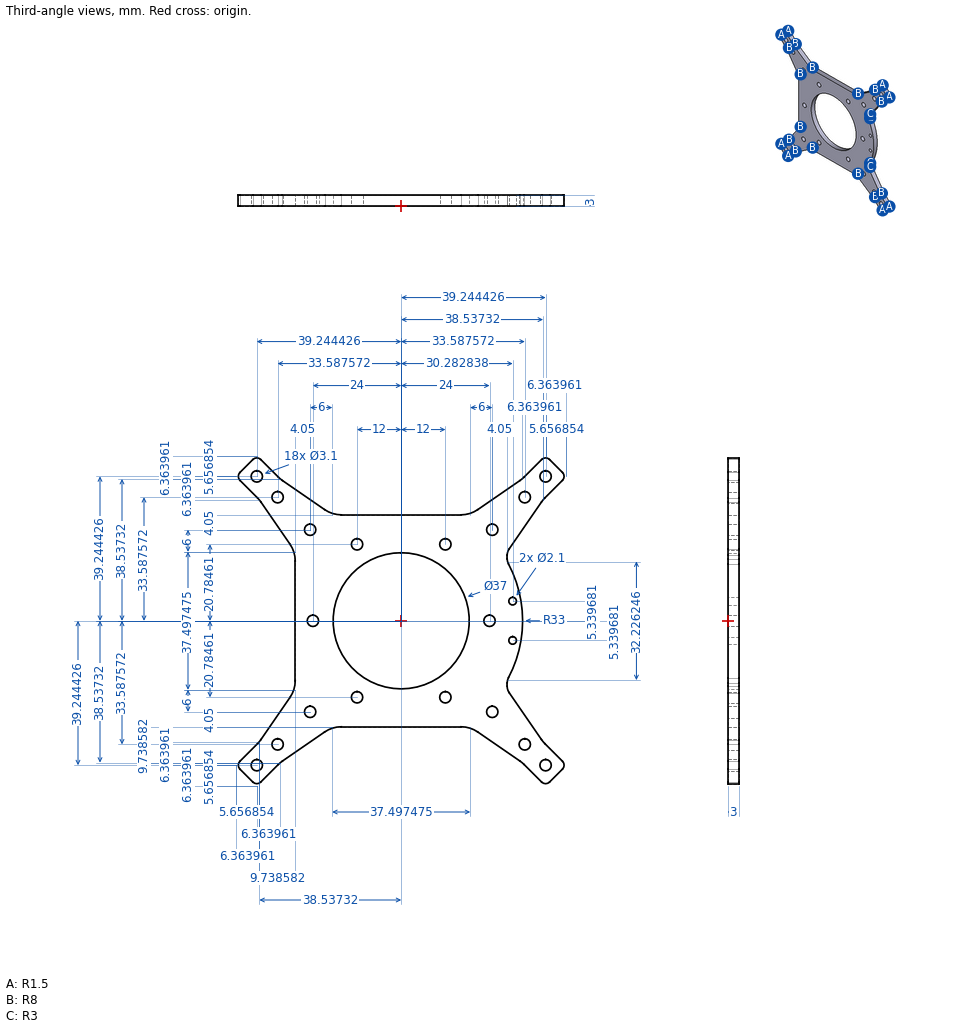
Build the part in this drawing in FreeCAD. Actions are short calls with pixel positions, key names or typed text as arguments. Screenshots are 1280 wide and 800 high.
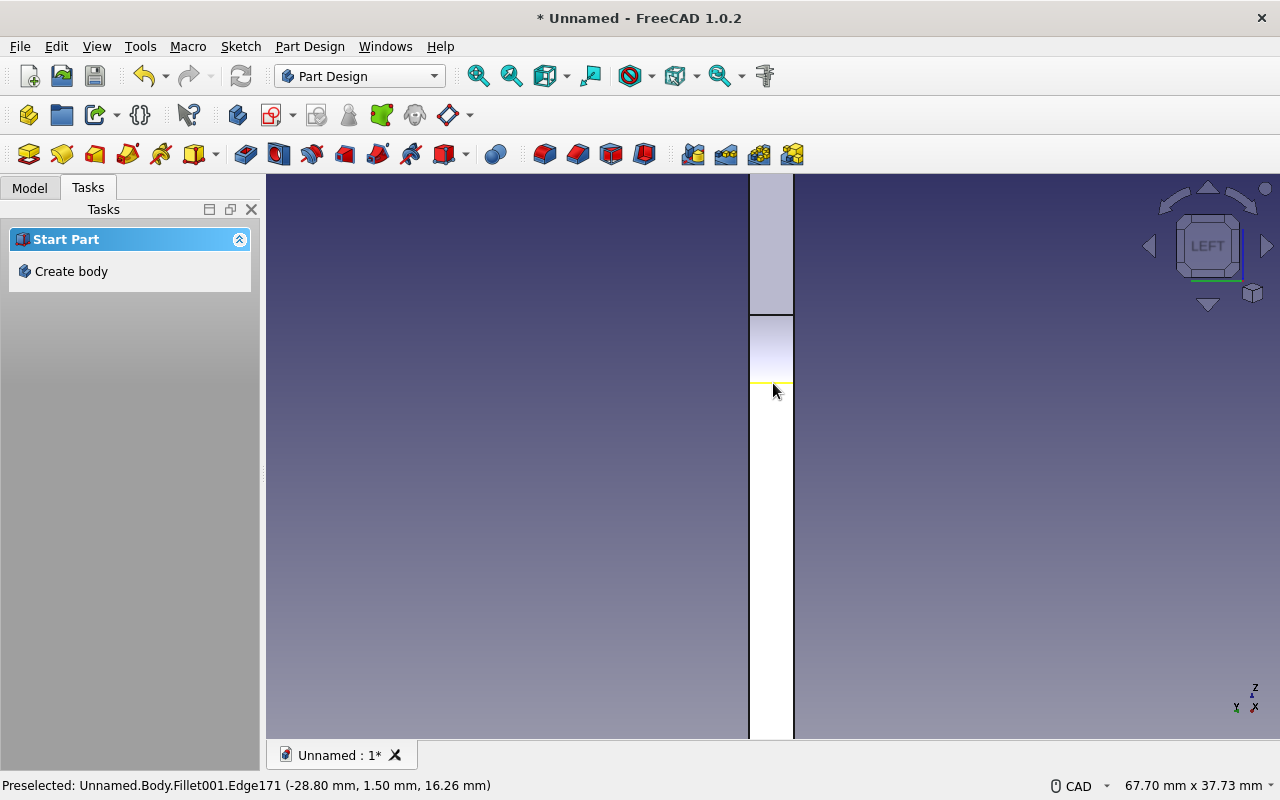
click(479, 76)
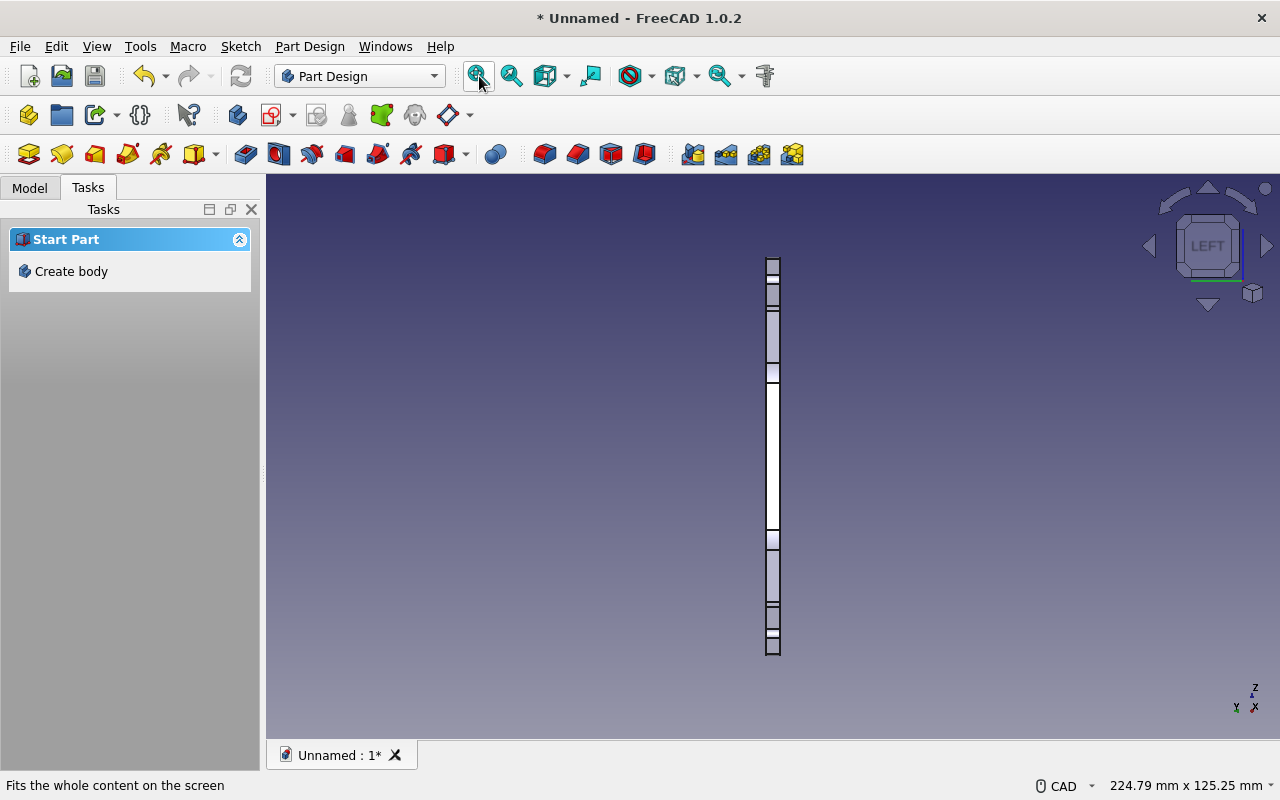
key(0)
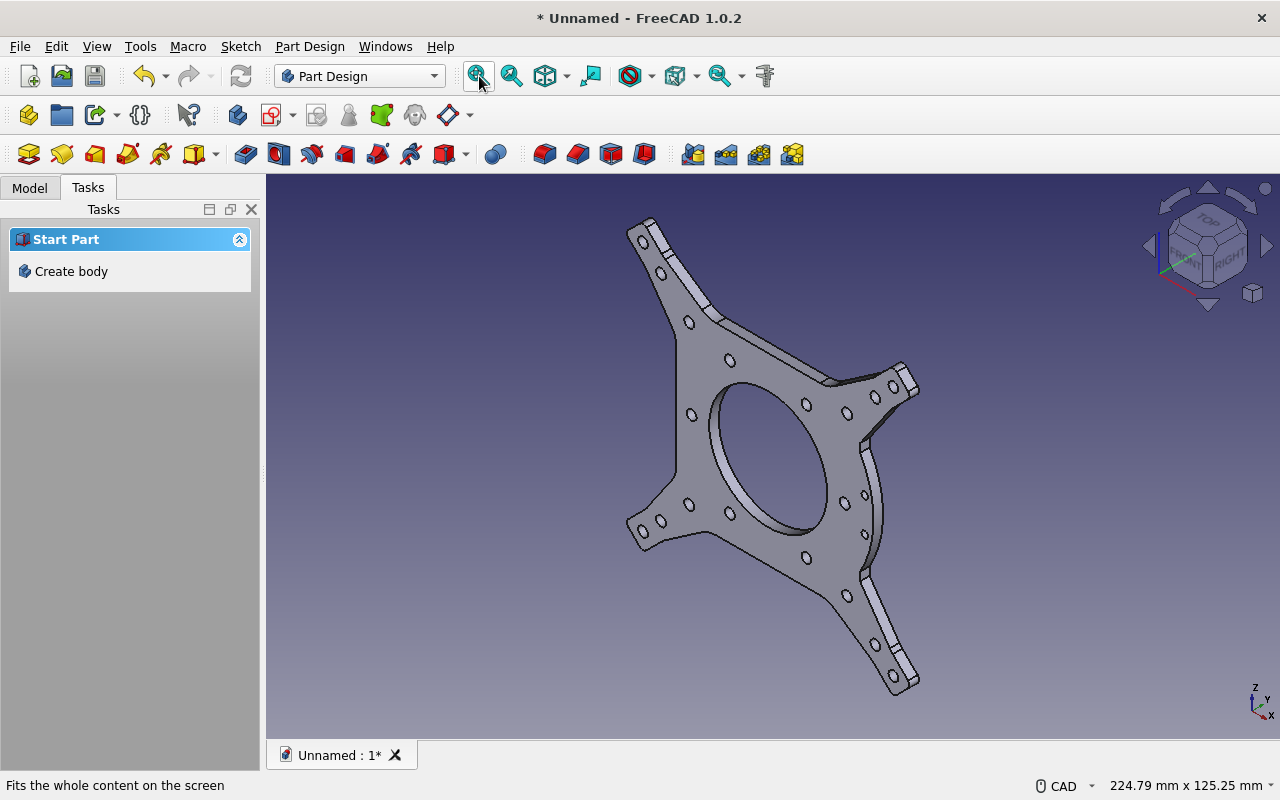
scroll(865, 449, up, 6)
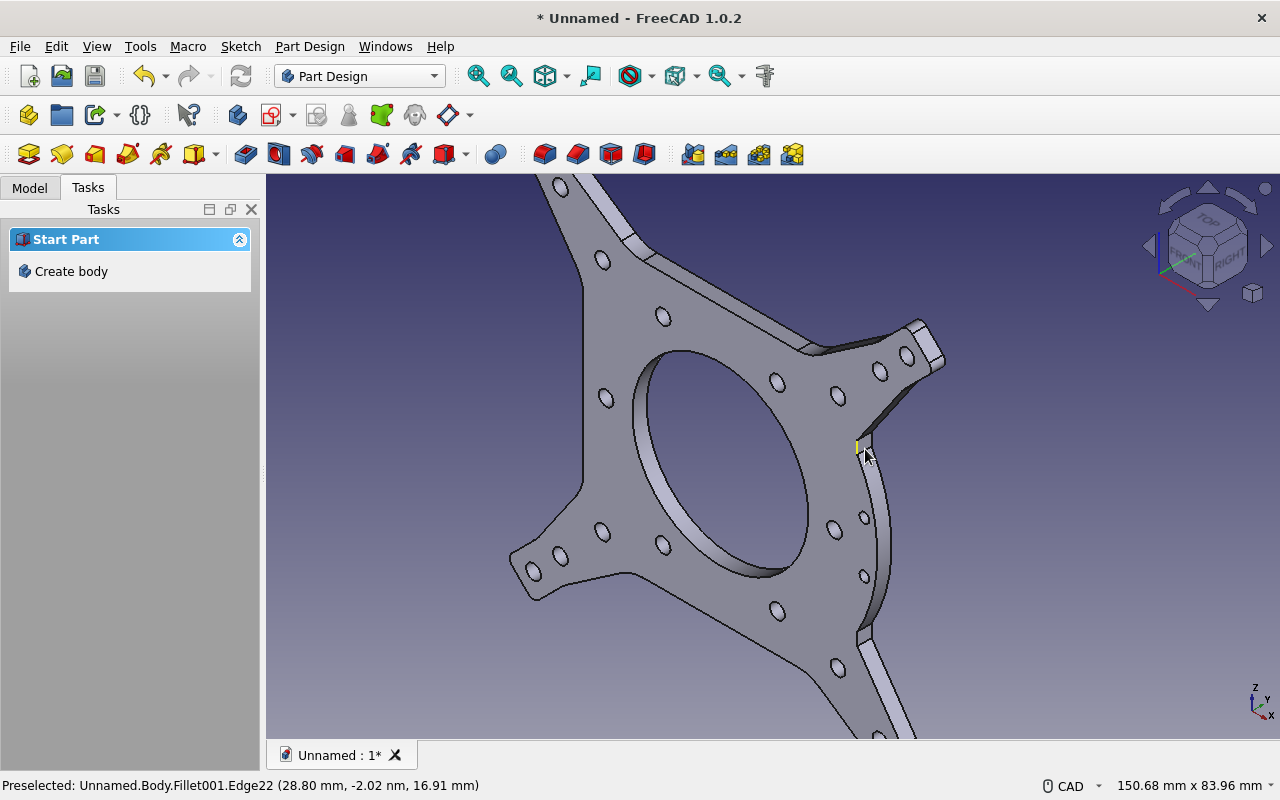
key(v)
key(f)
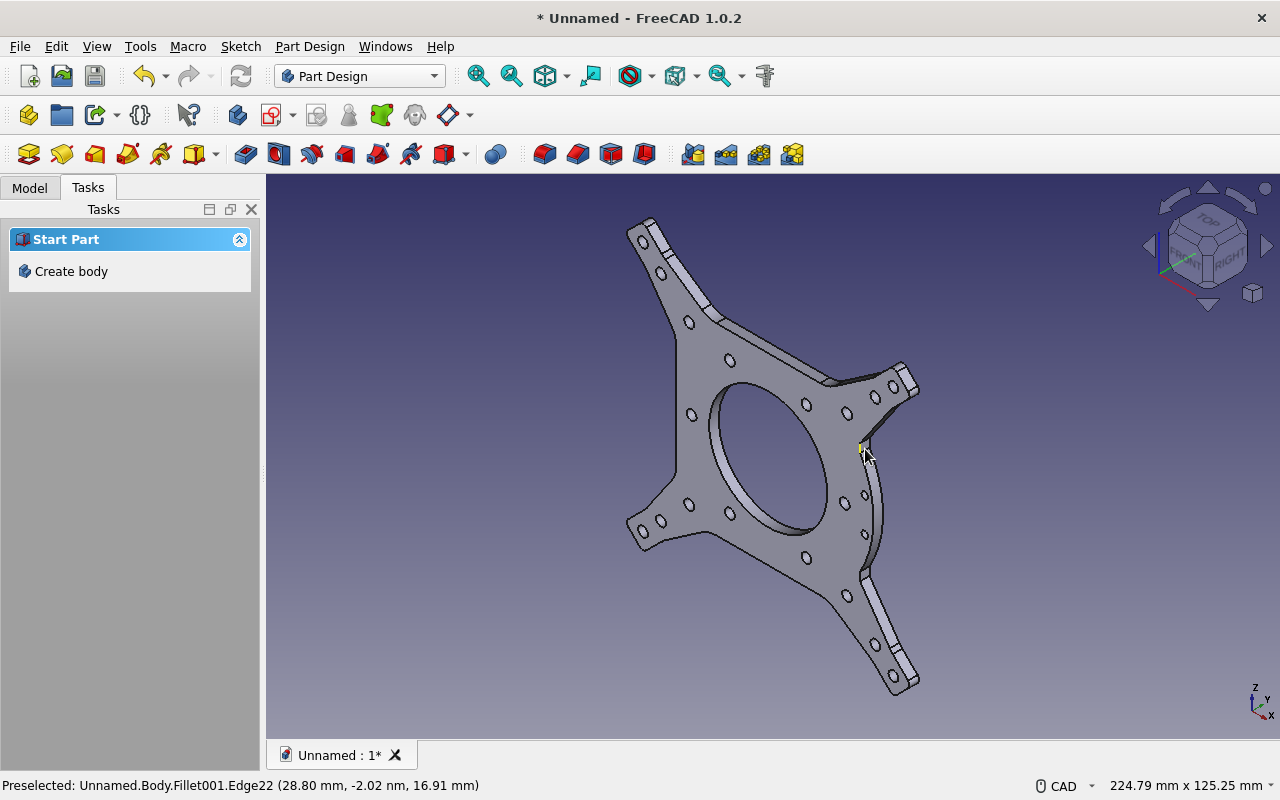
key(2)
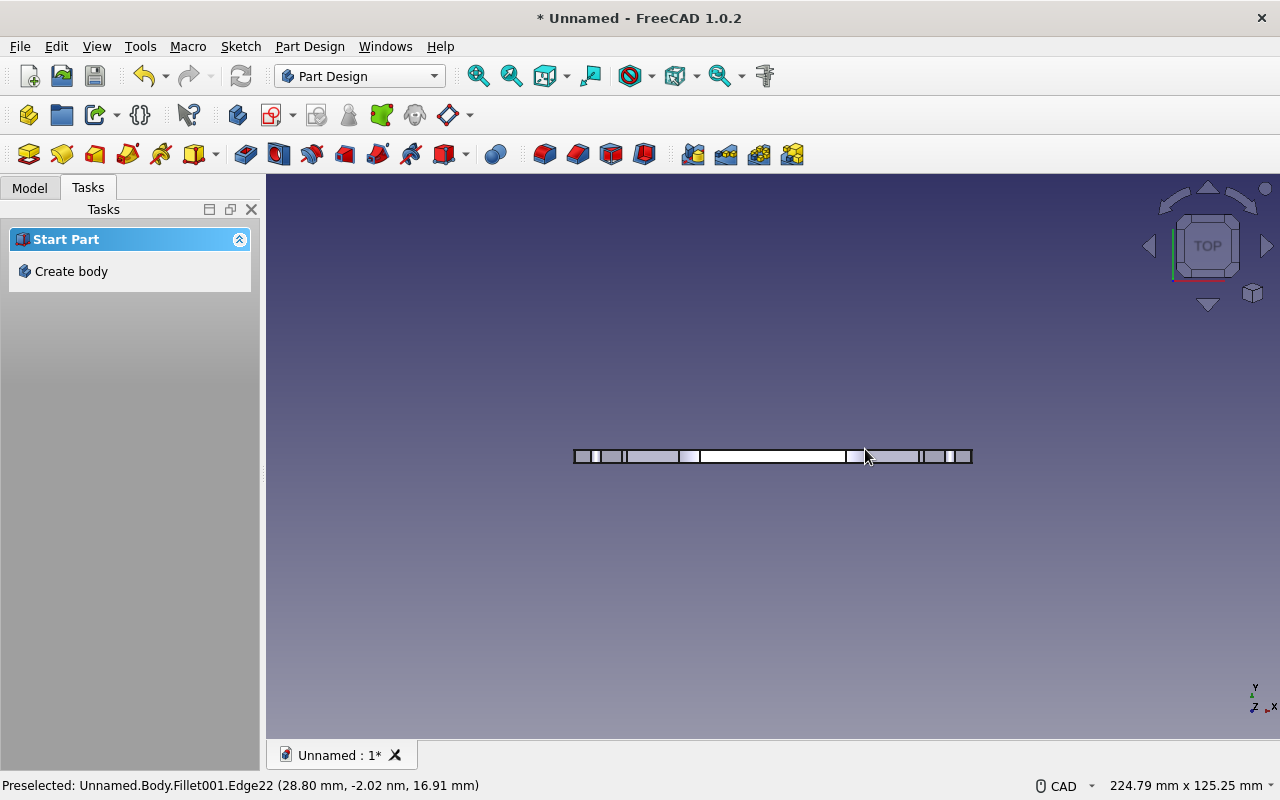
click(479, 76)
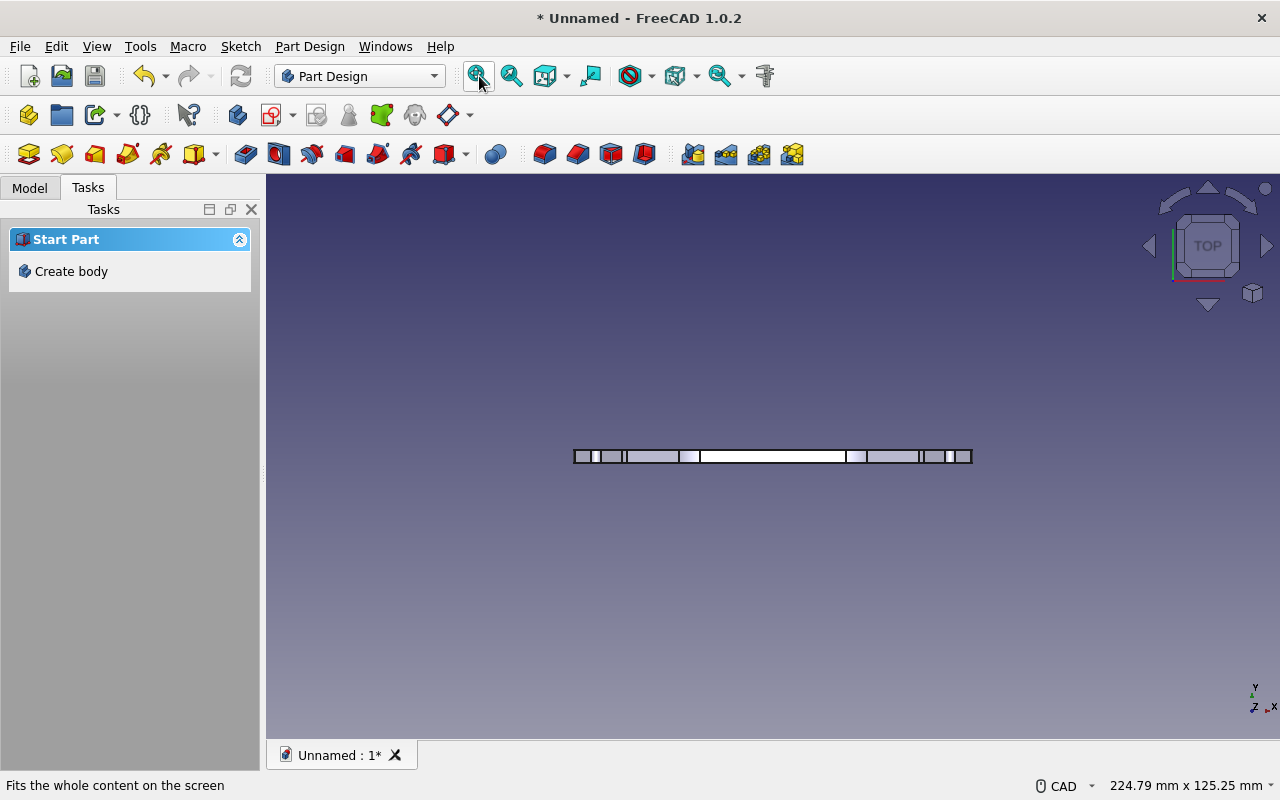
scroll(903, 455, up, 6)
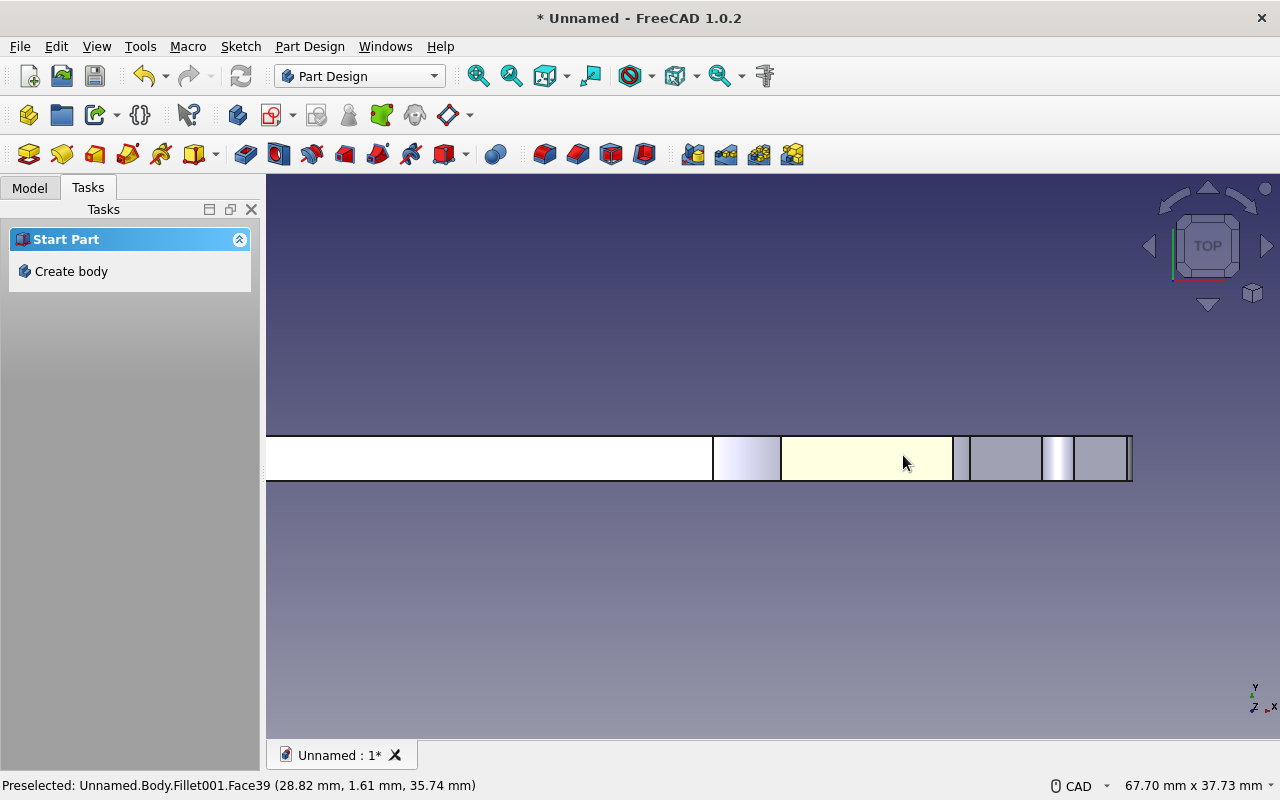
click(479, 76)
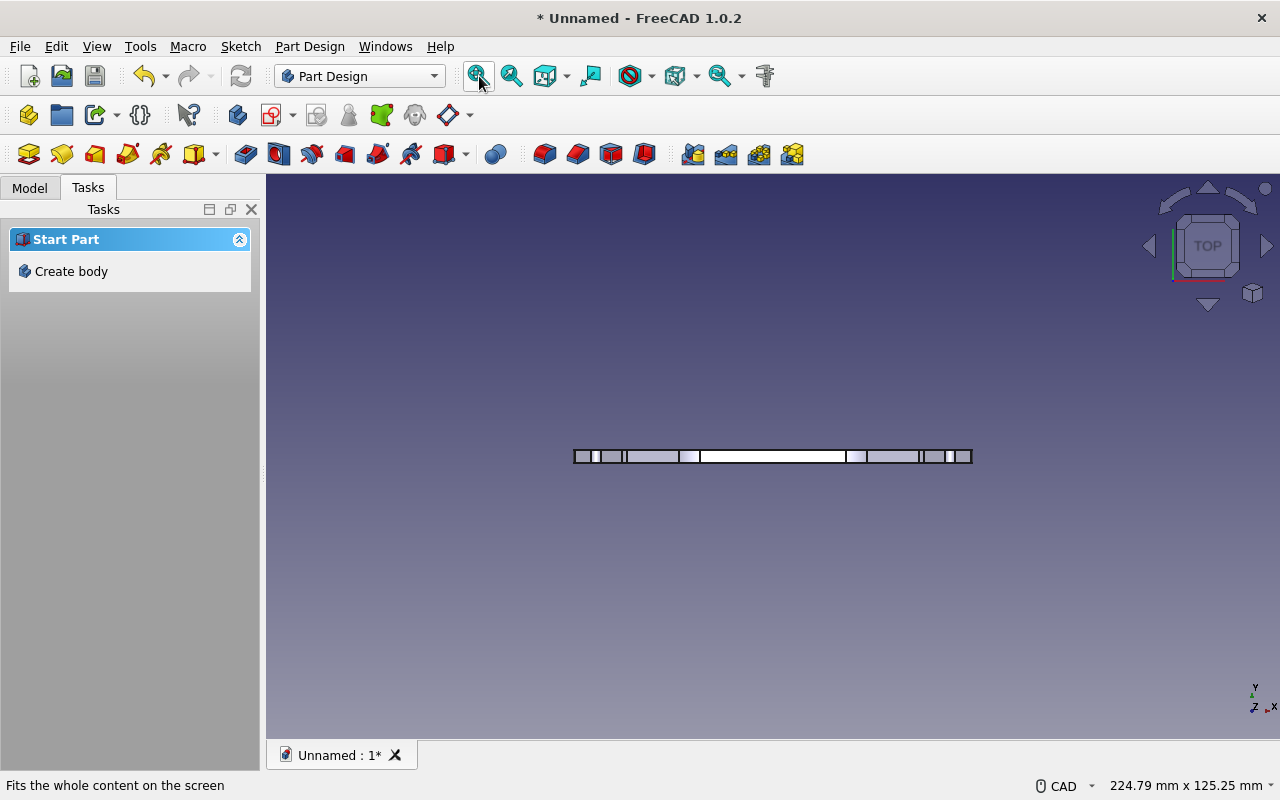
key(1)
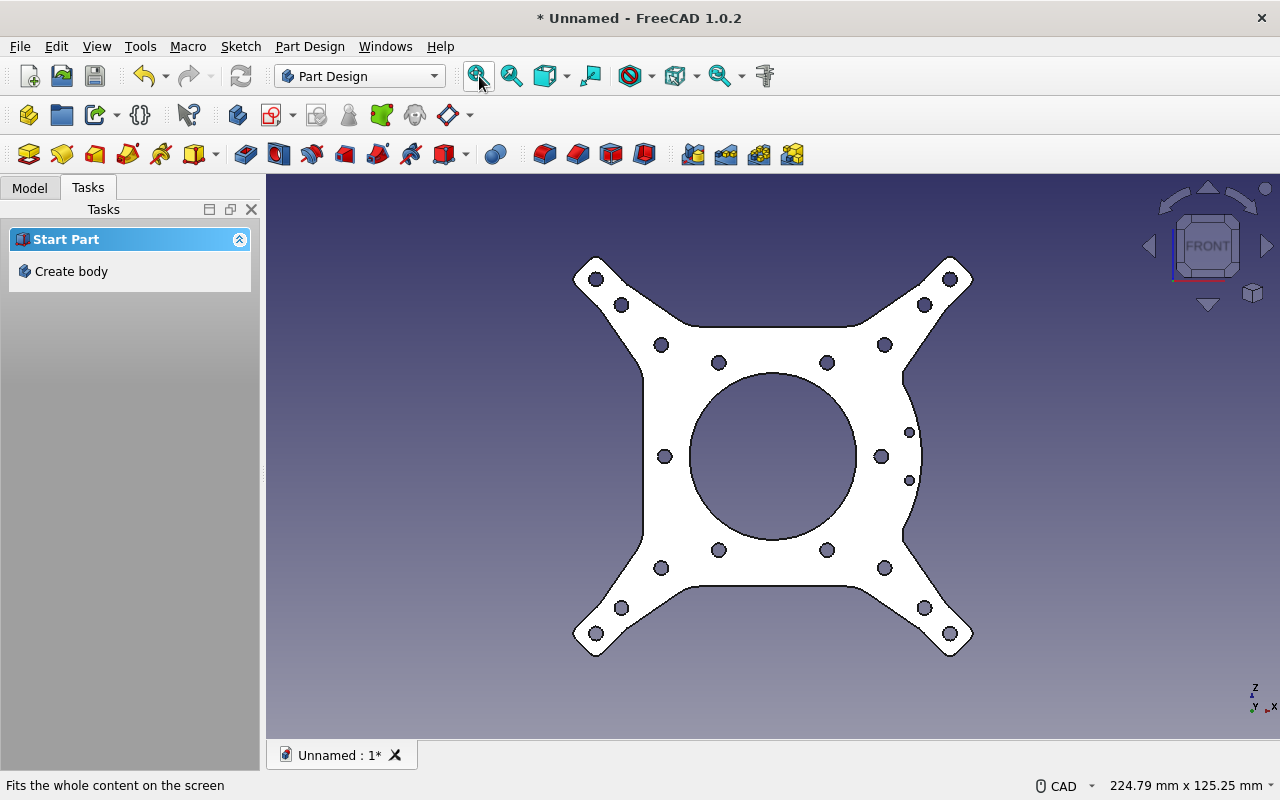
scroll(903, 383, up, 6)